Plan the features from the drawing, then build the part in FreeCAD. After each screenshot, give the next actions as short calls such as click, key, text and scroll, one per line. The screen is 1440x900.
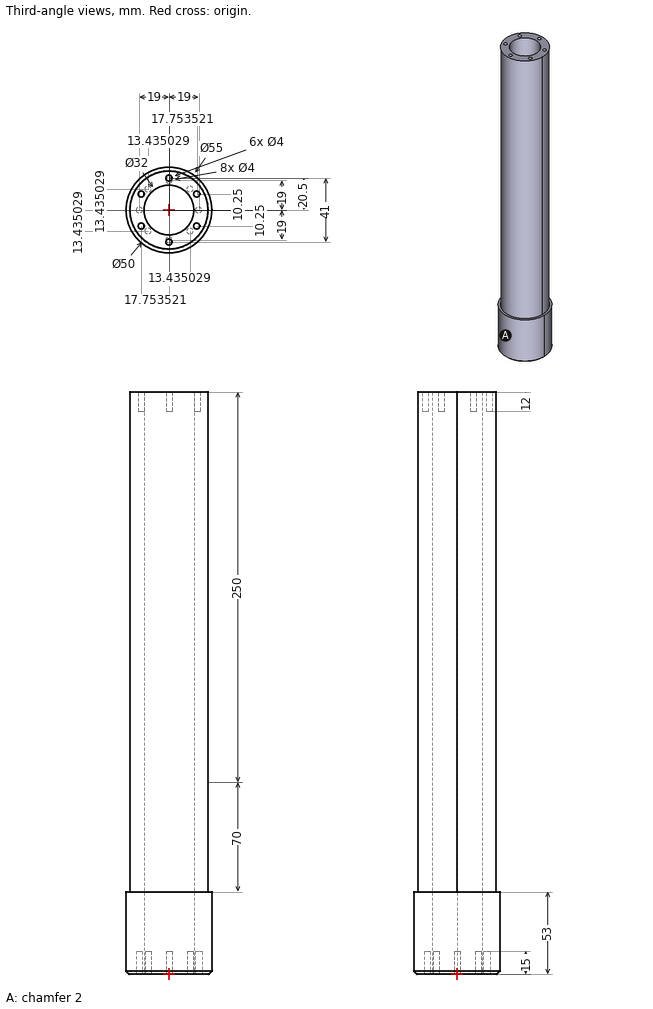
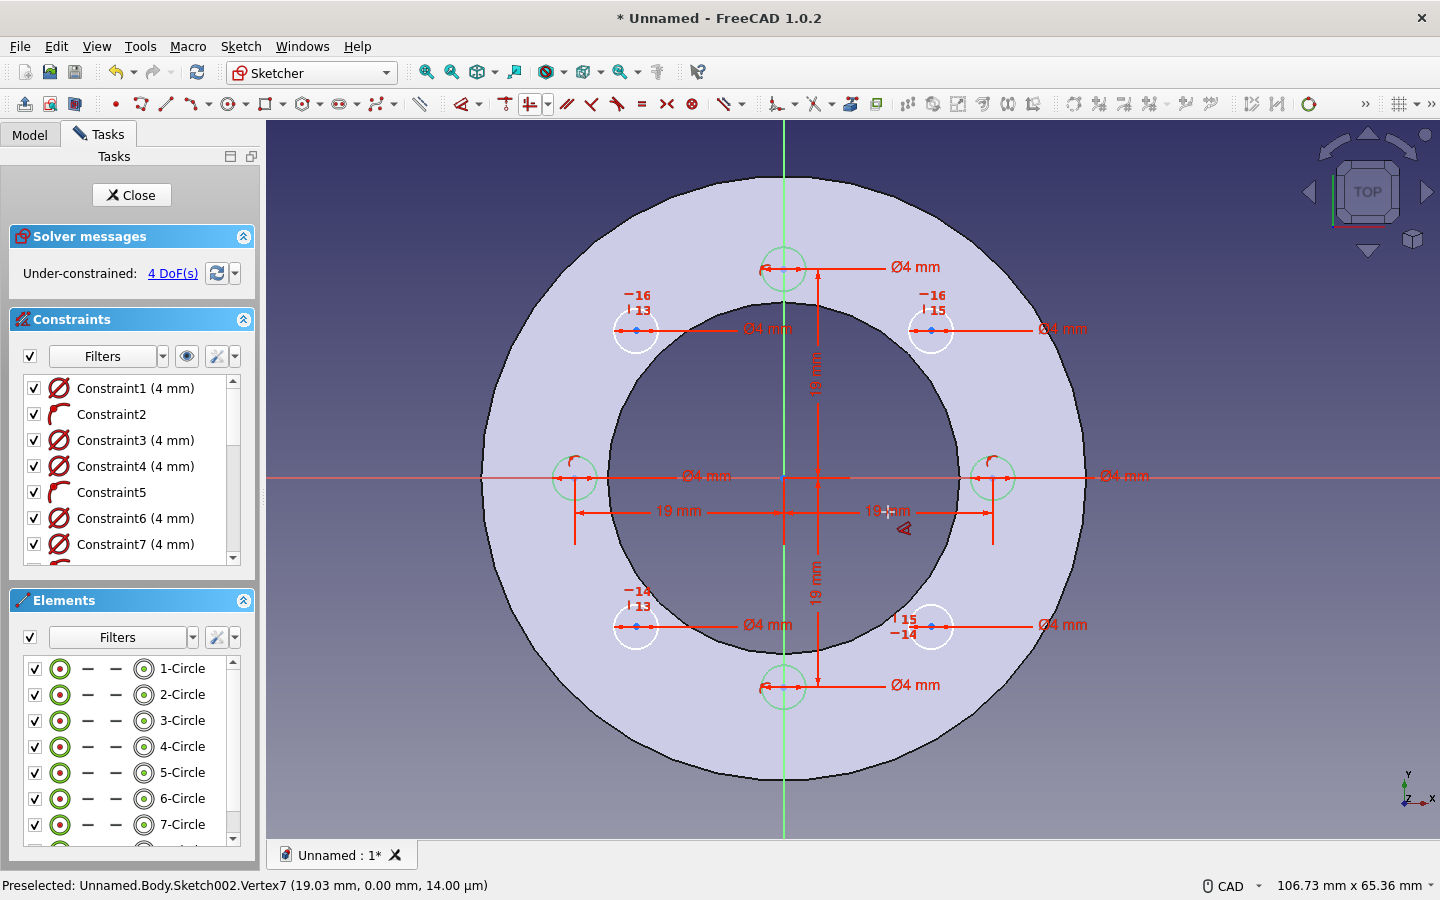
click(636, 331)
click(710, 297)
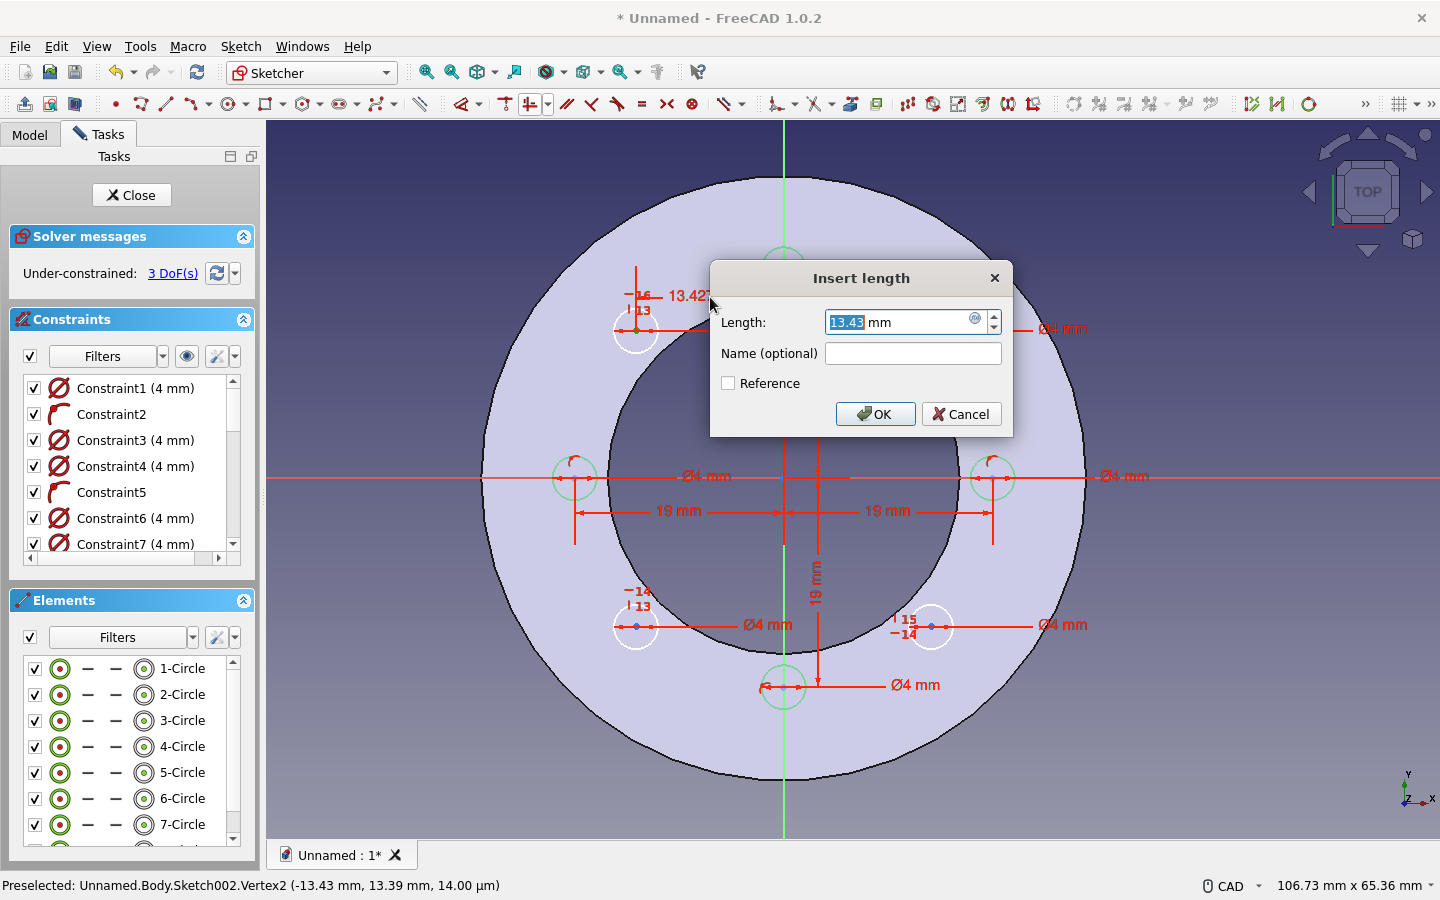
text(13.435029)
key(Return)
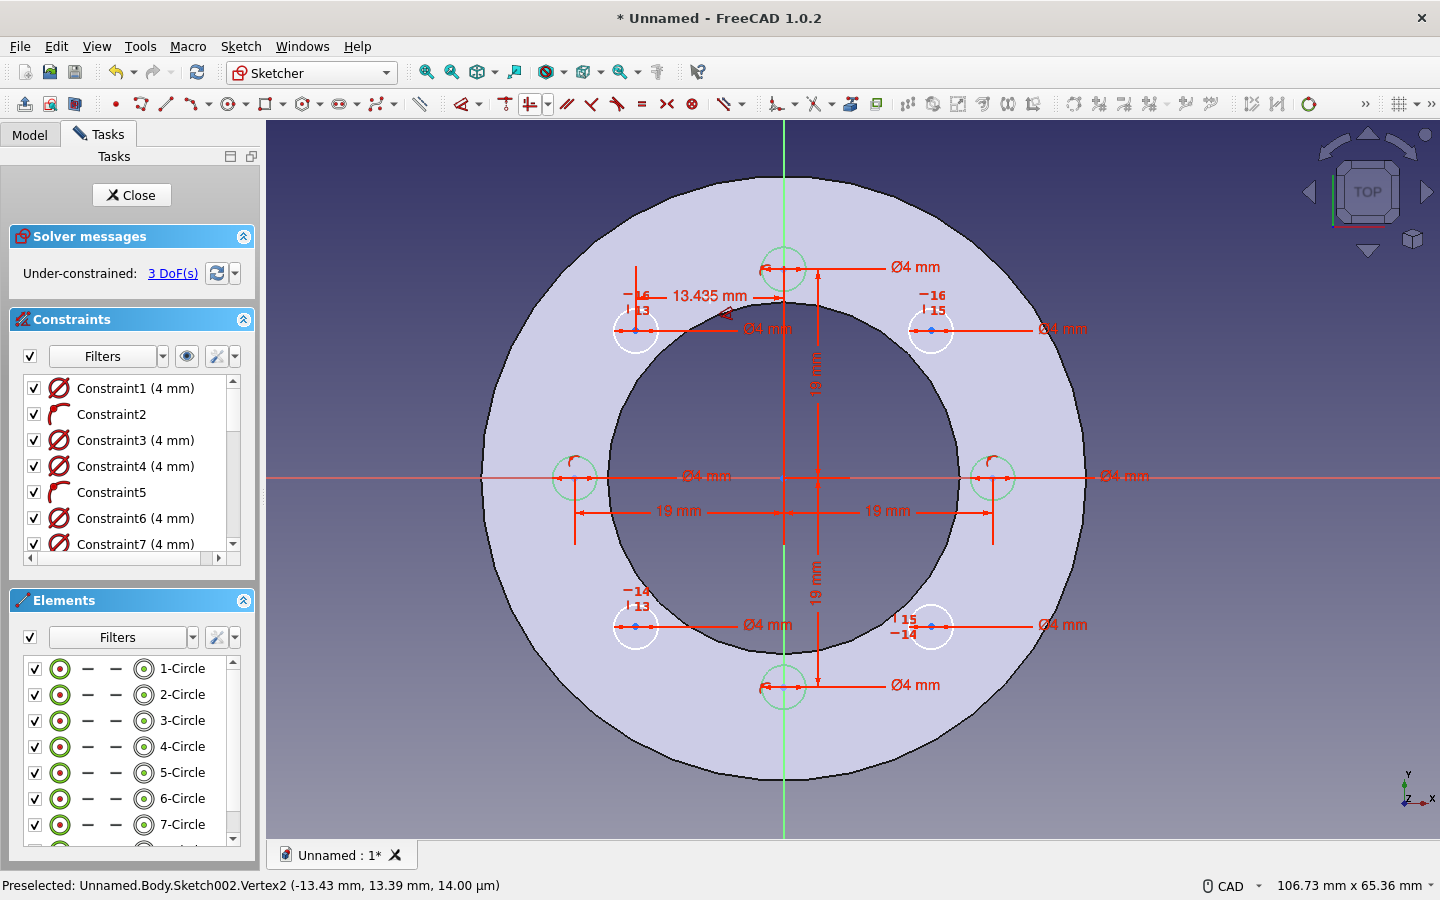
click(636, 331)
click(602, 405)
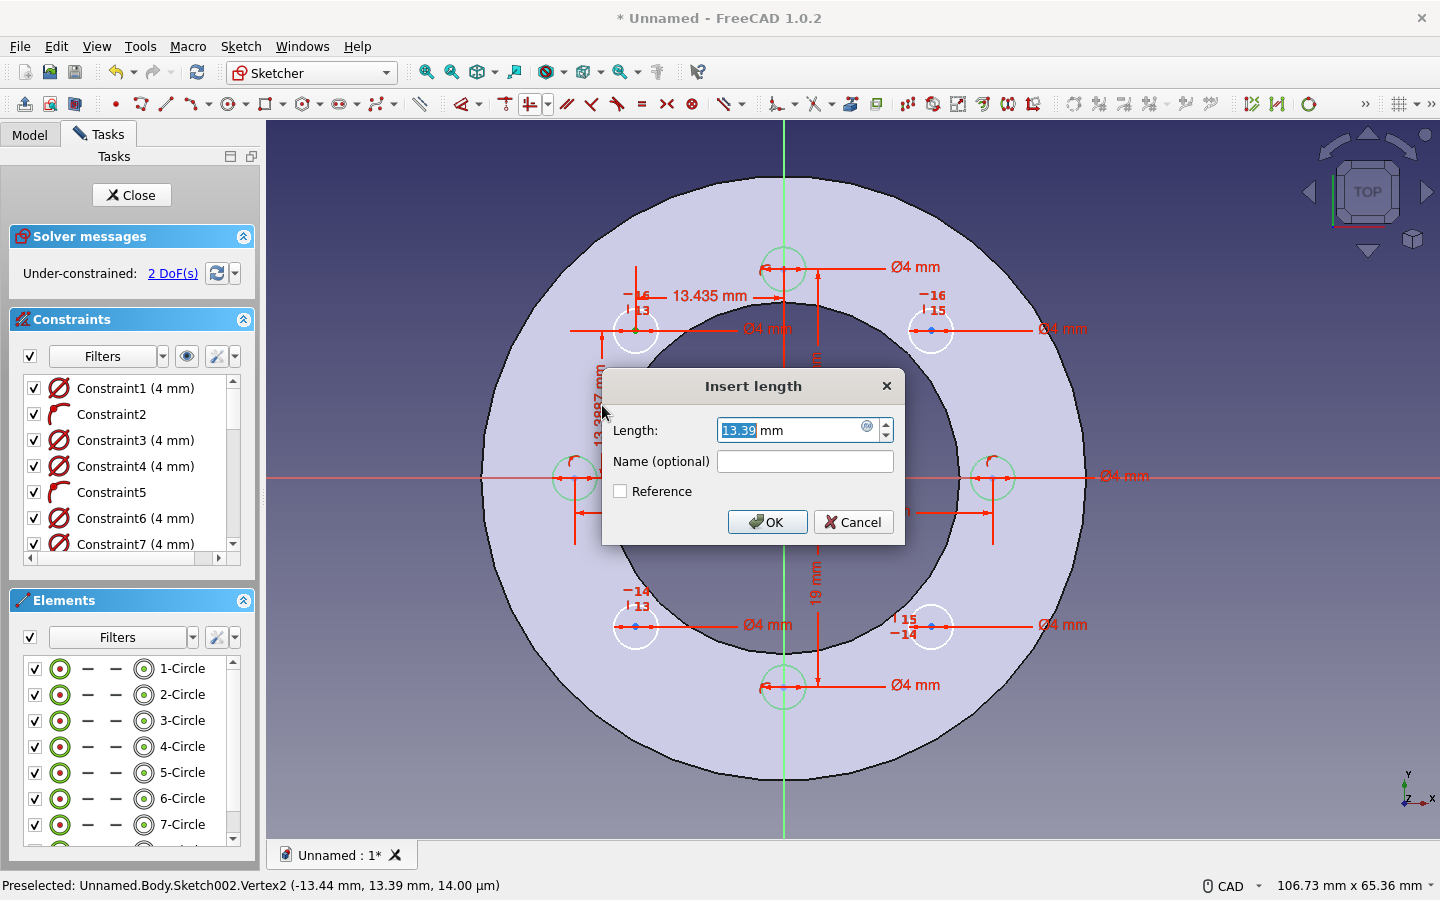
text(13.435029)
key(Return)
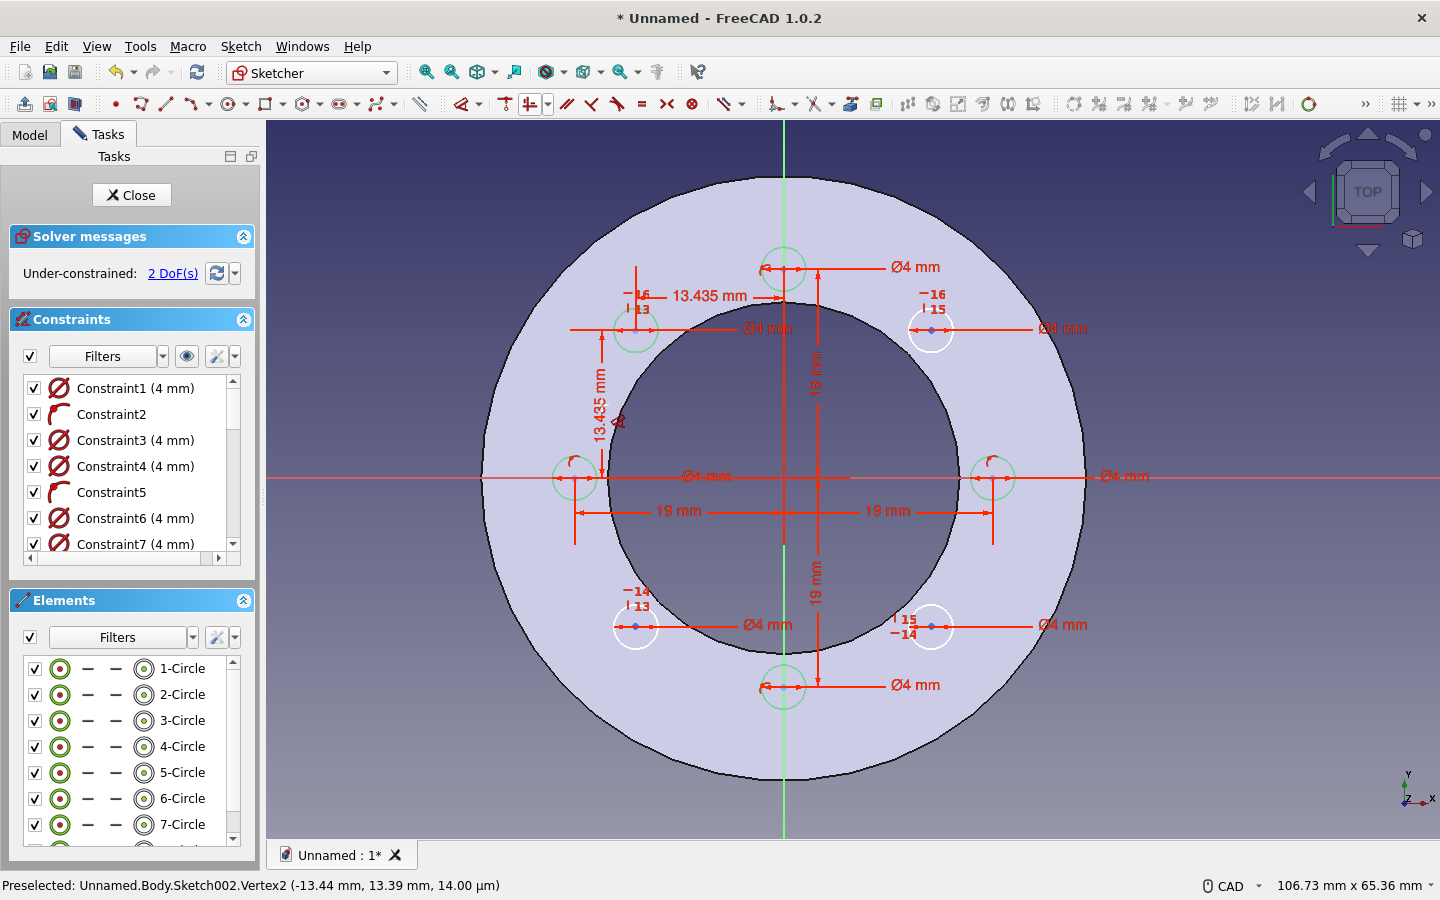
click(636, 627)
click(602, 553)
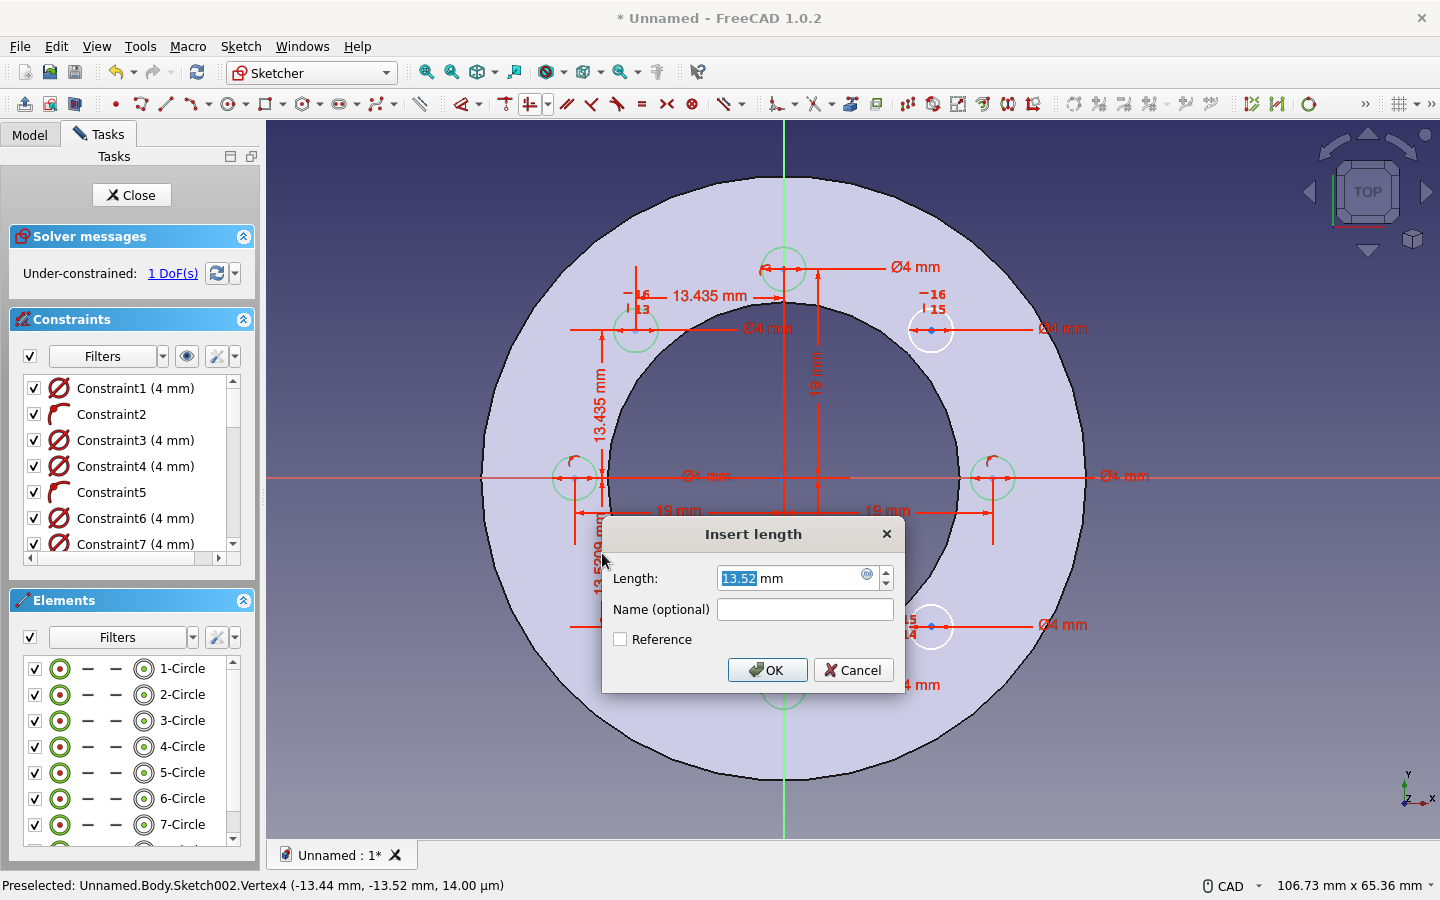
text(13.435029)
key(Return)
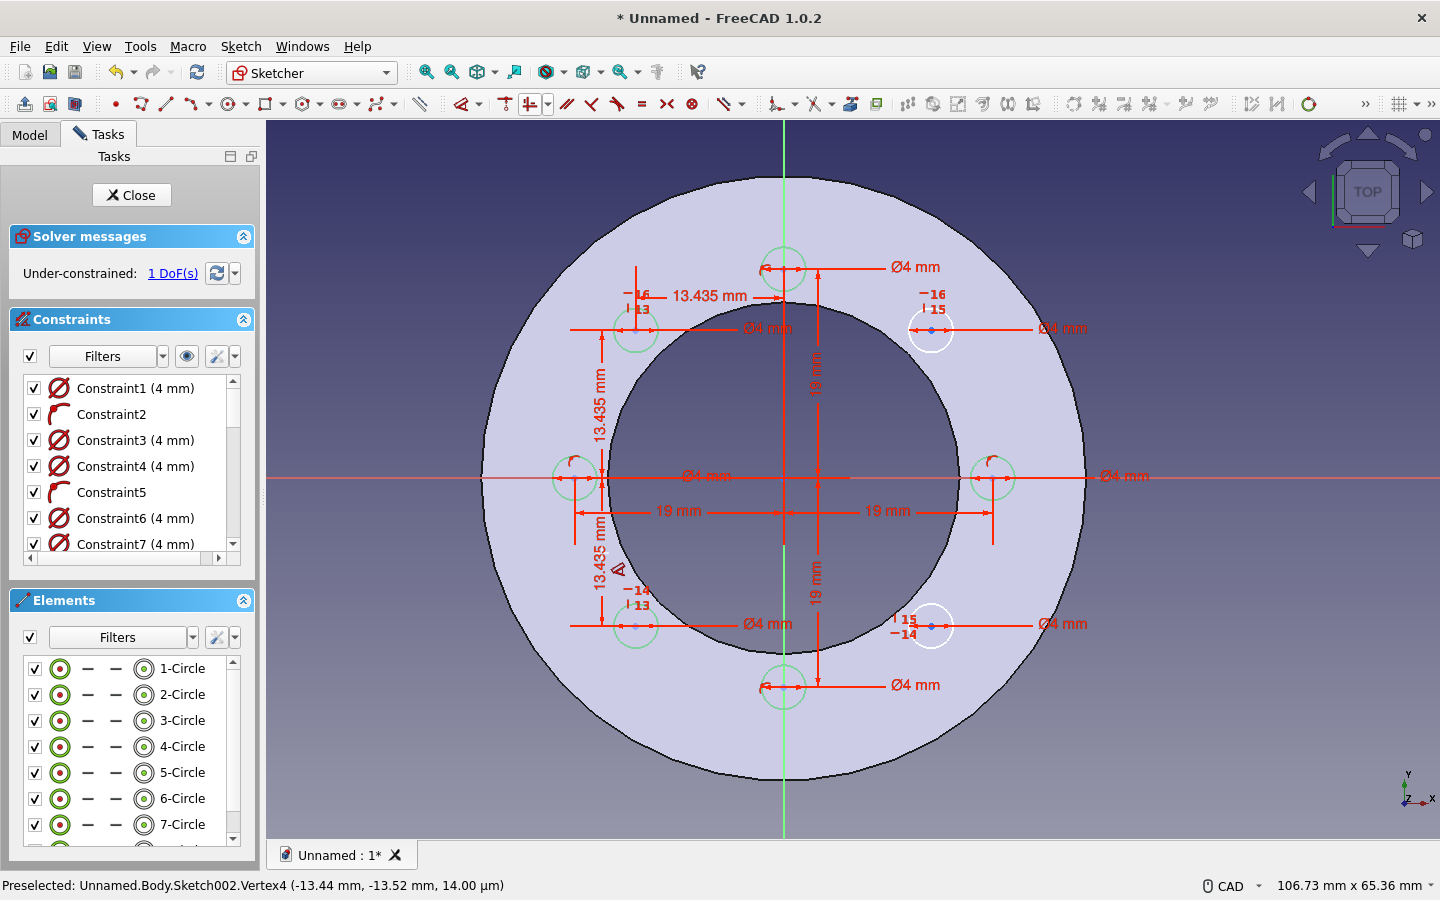
click(931, 626)
click(857, 660)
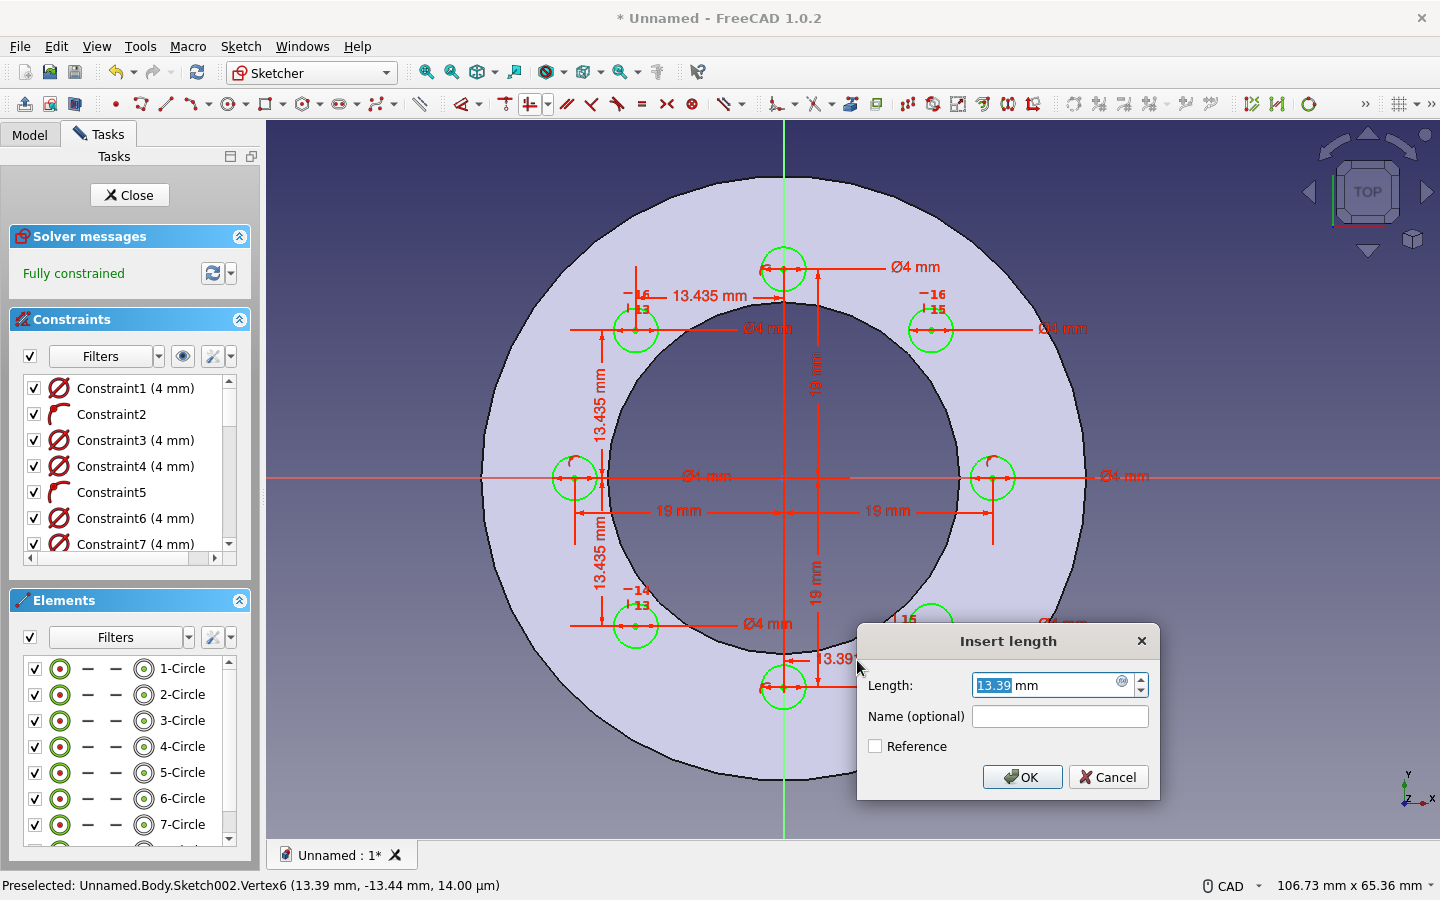
text(13.435029)
key(Return)
key(Escape)